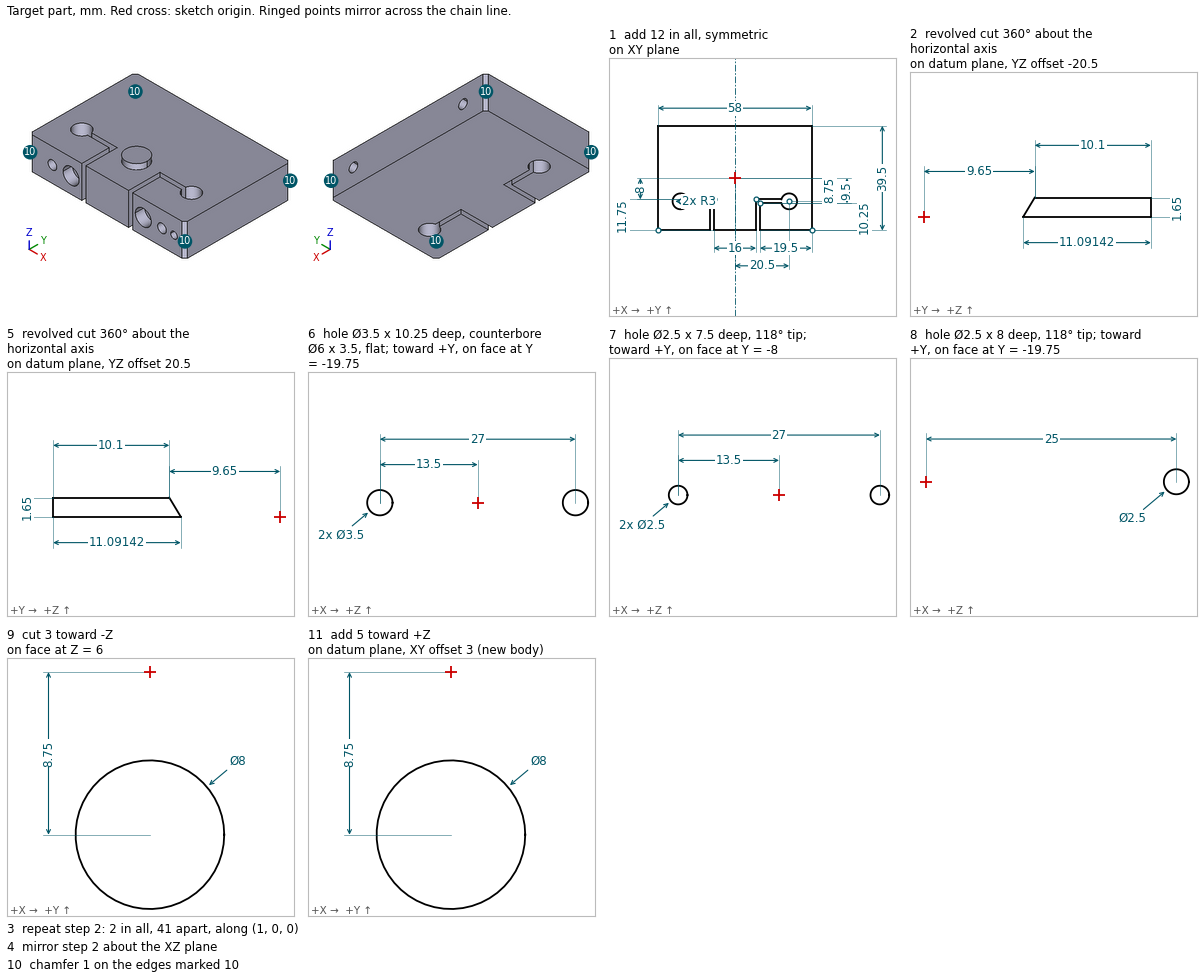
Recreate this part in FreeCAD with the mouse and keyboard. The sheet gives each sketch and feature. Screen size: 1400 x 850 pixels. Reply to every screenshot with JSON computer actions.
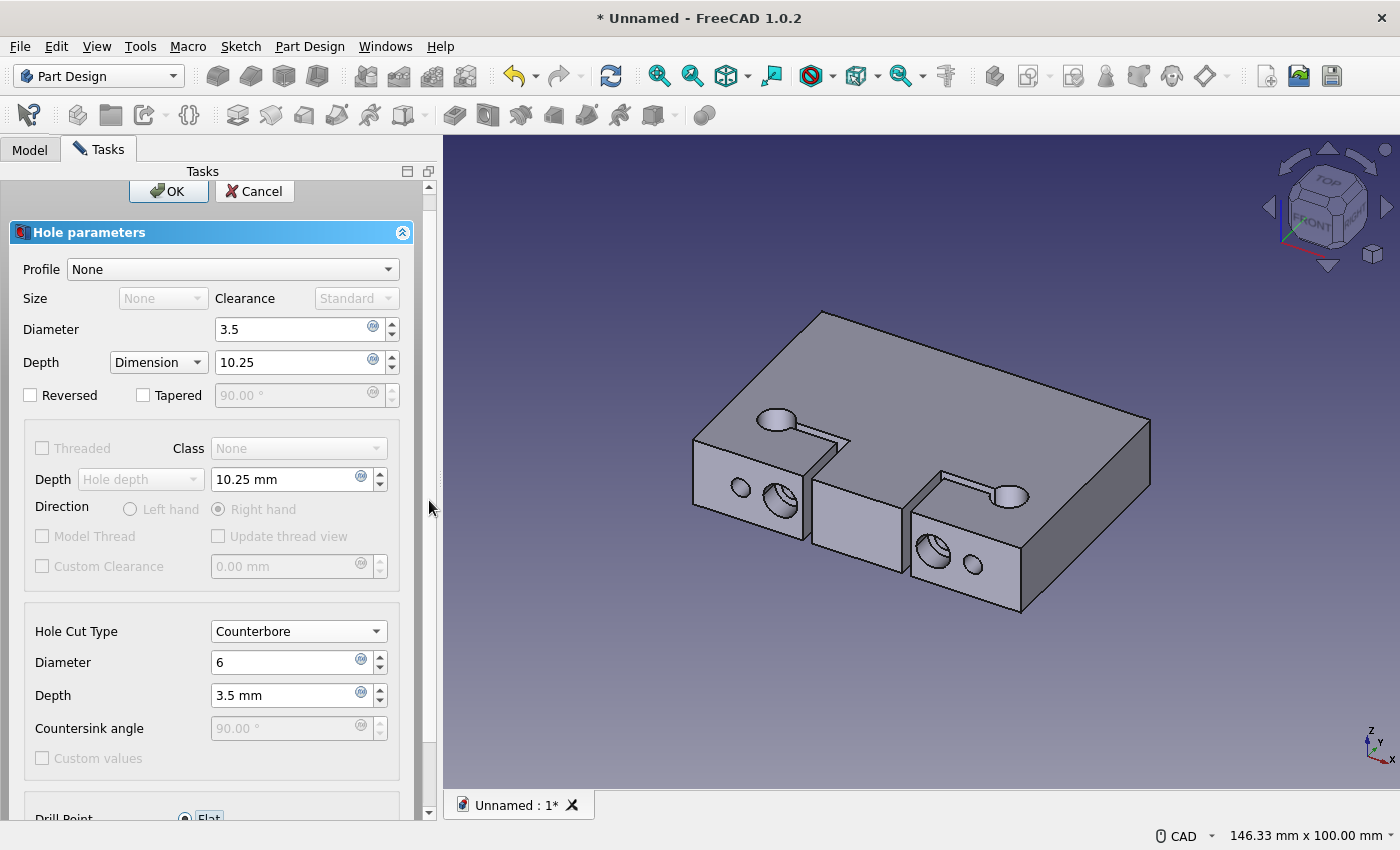
{"action": "left_click", "coordinate": [169, 210]}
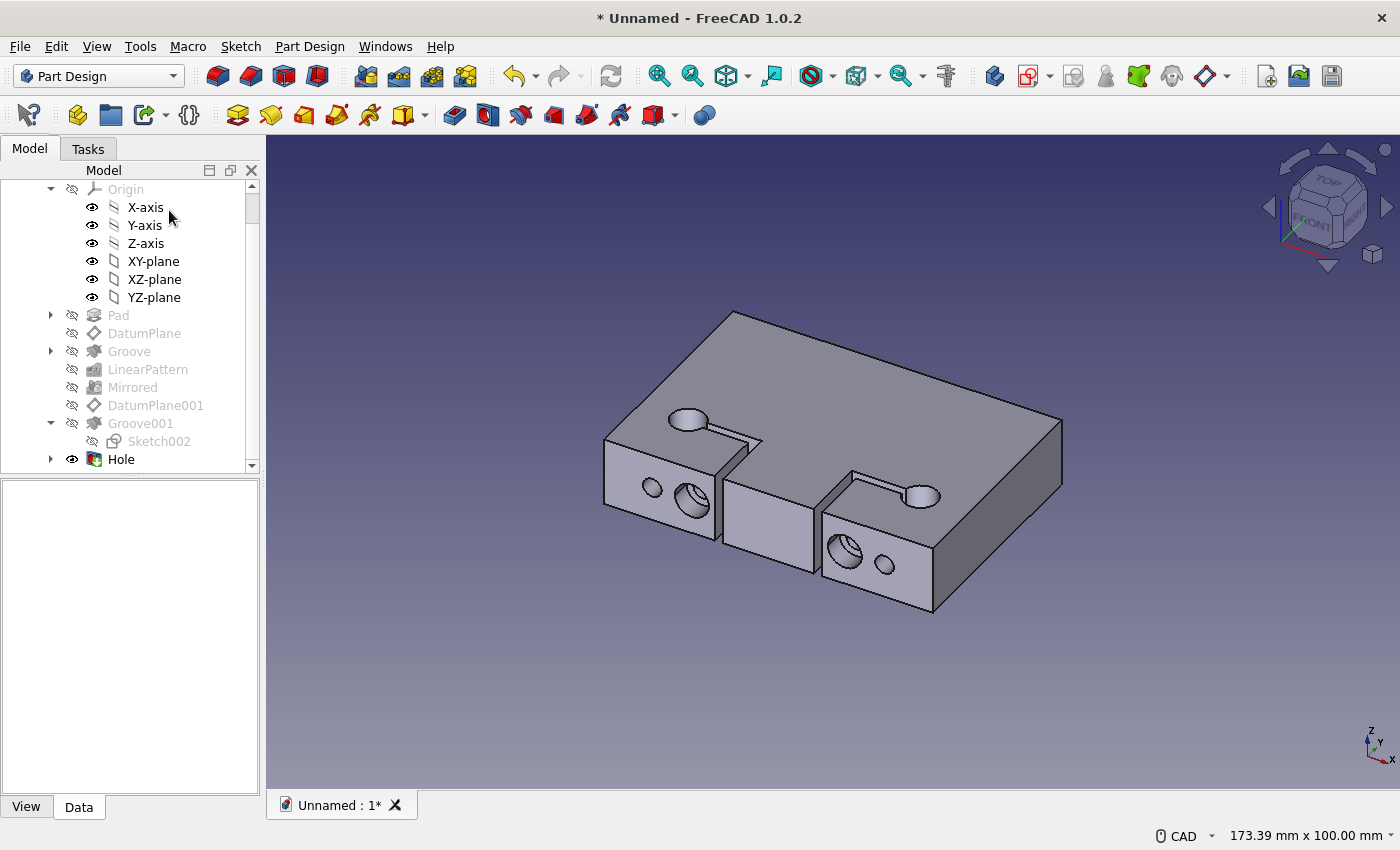
{"action": "key", "text": "0"}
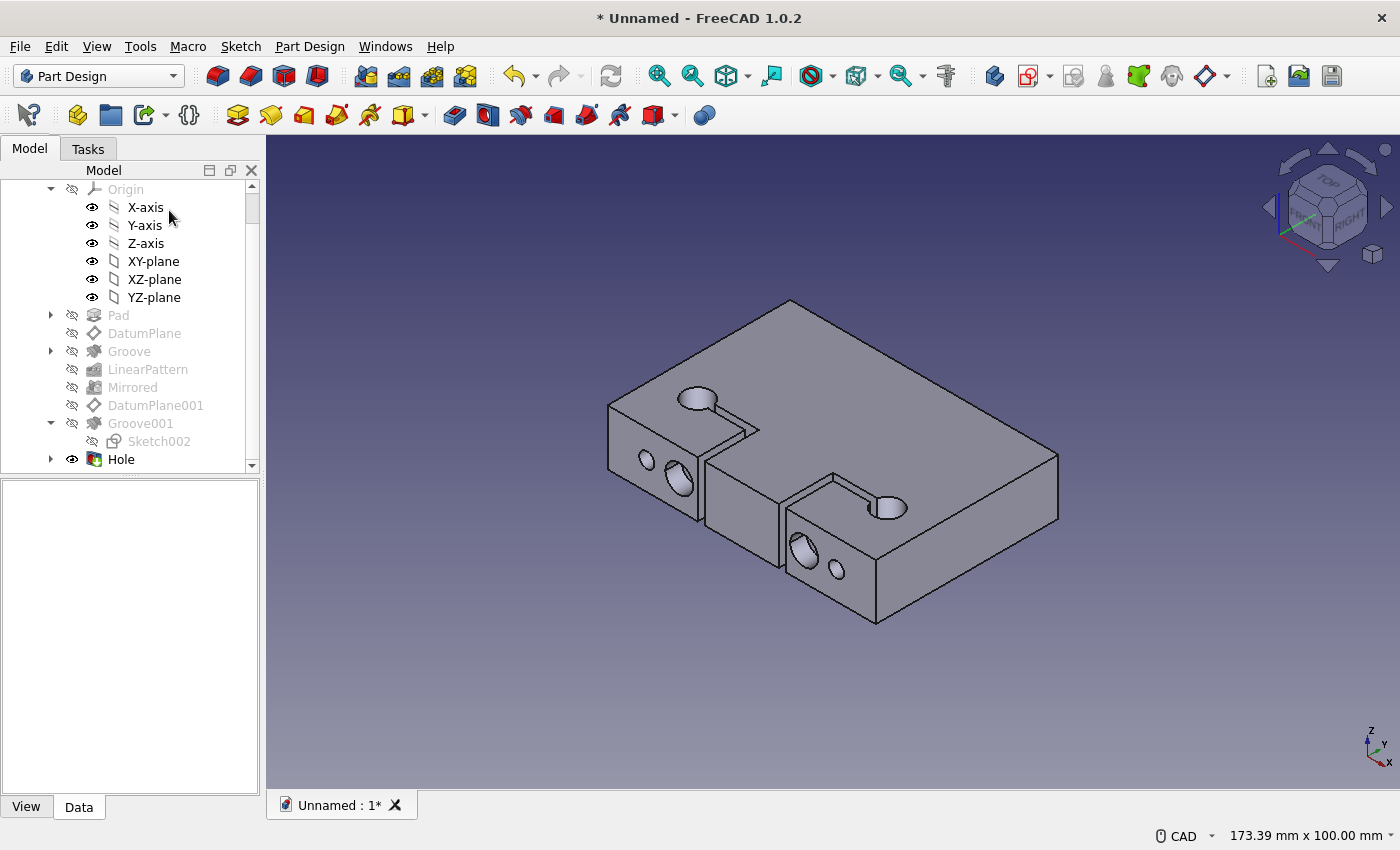
{"action": "key", "text": "1"}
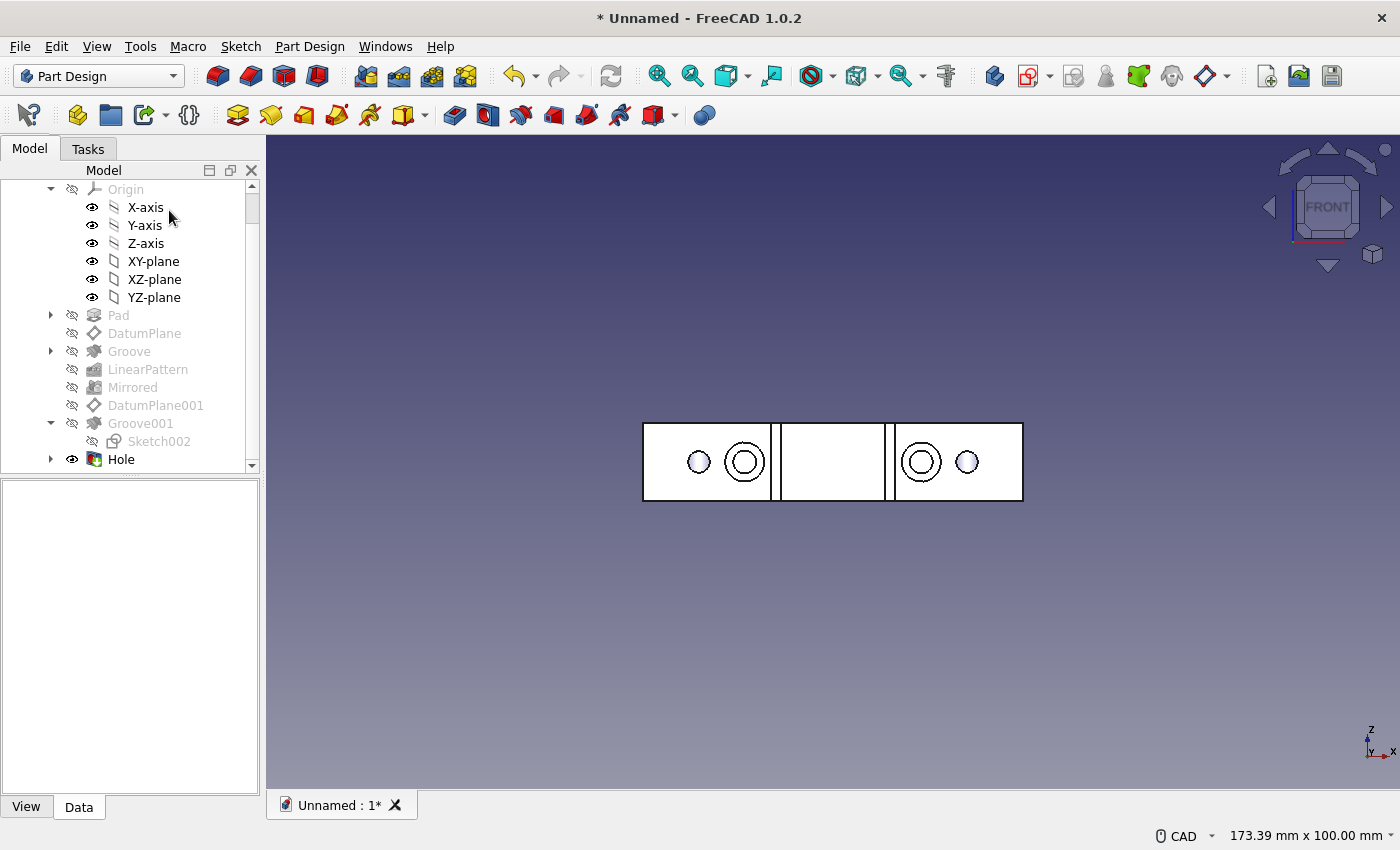
{"action": "left_click", "coordinate": [660, 76]}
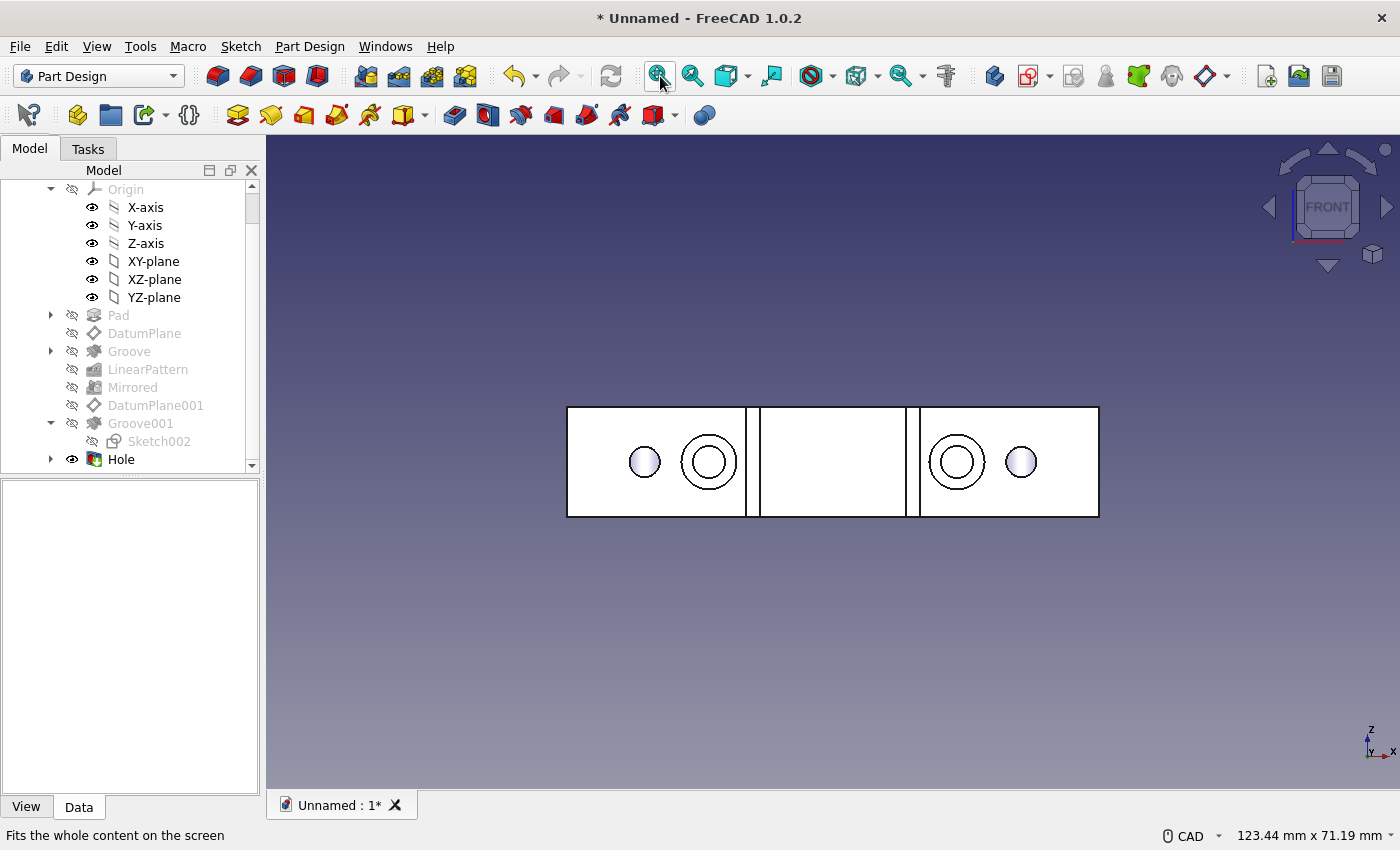
{"action": "left_click", "coordinate": [951, 461]}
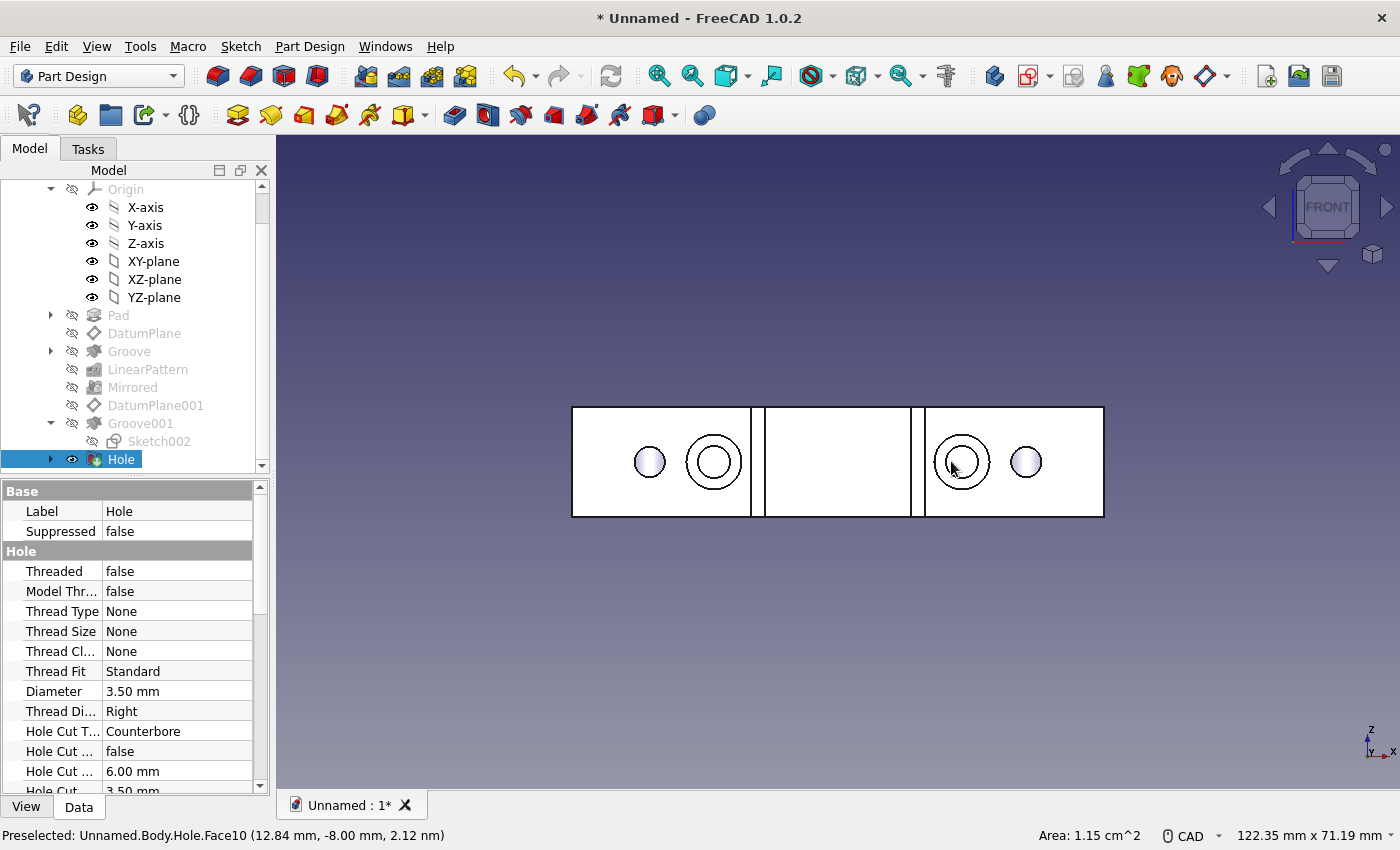
{"action": "left_click", "coordinate": [1028, 76]}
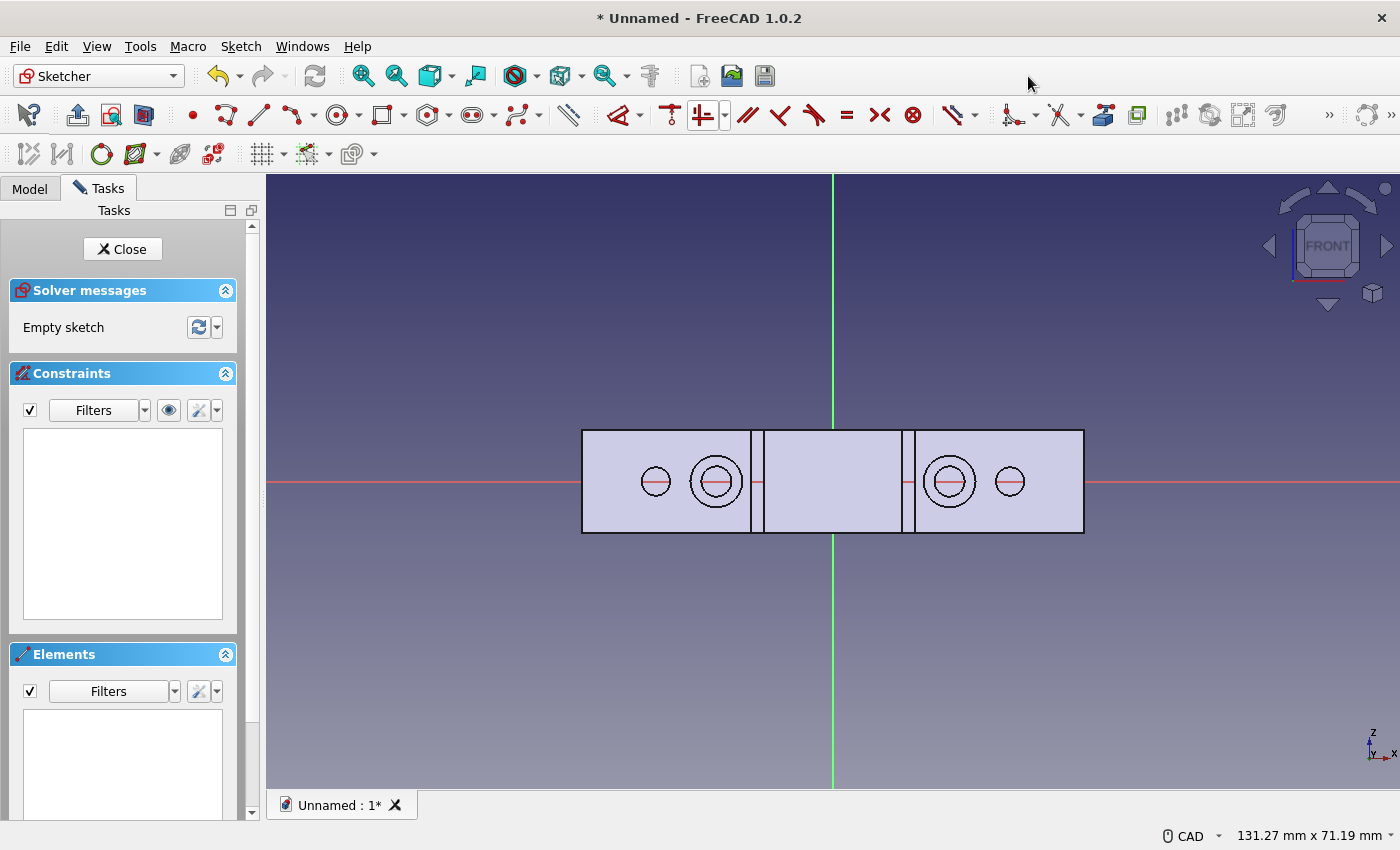
{"action": "scroll", "coordinate": [873, 482], "scroll_direction": "up", "scroll_amount": 5}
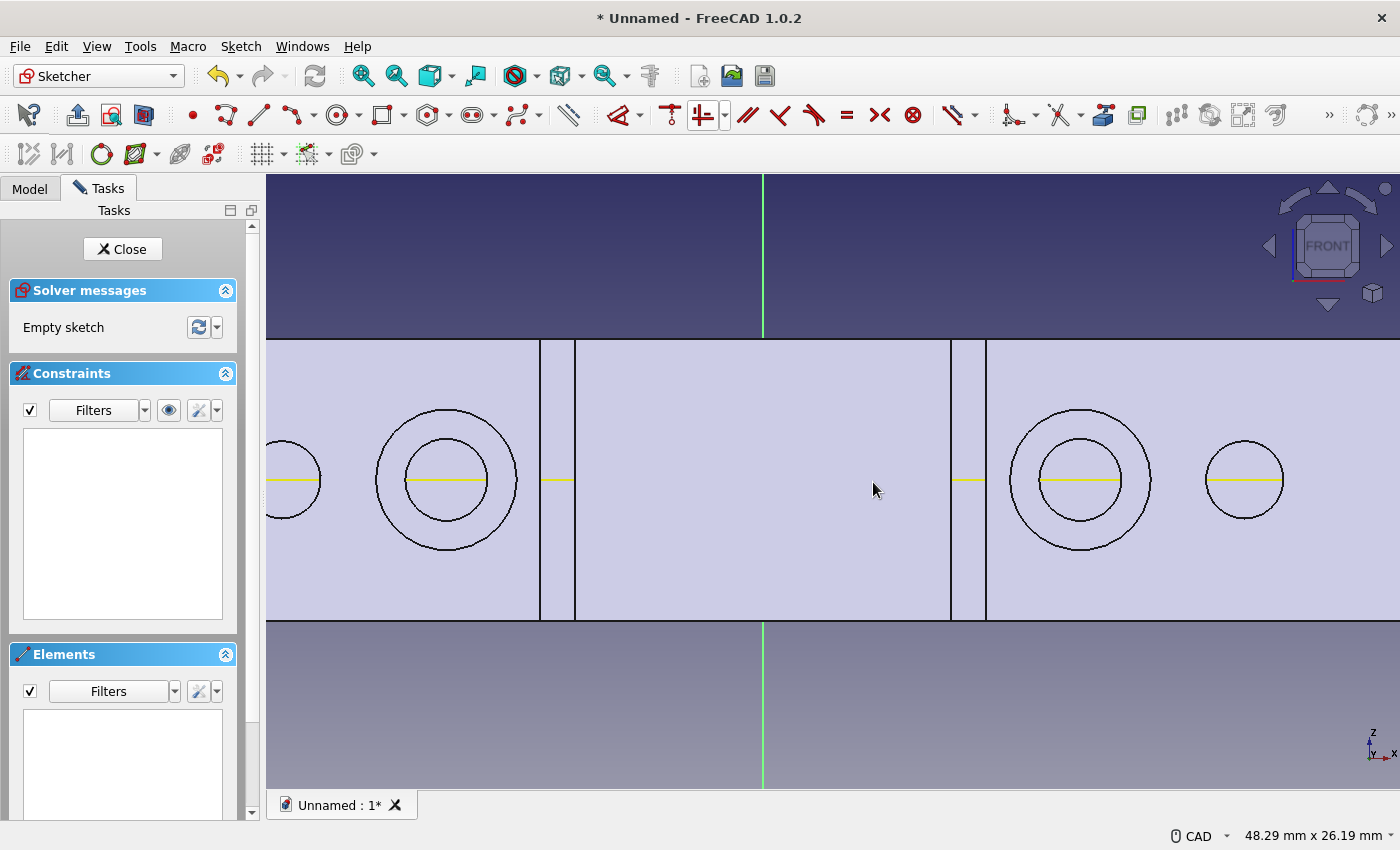
{"action": "key", "text": "g c"}